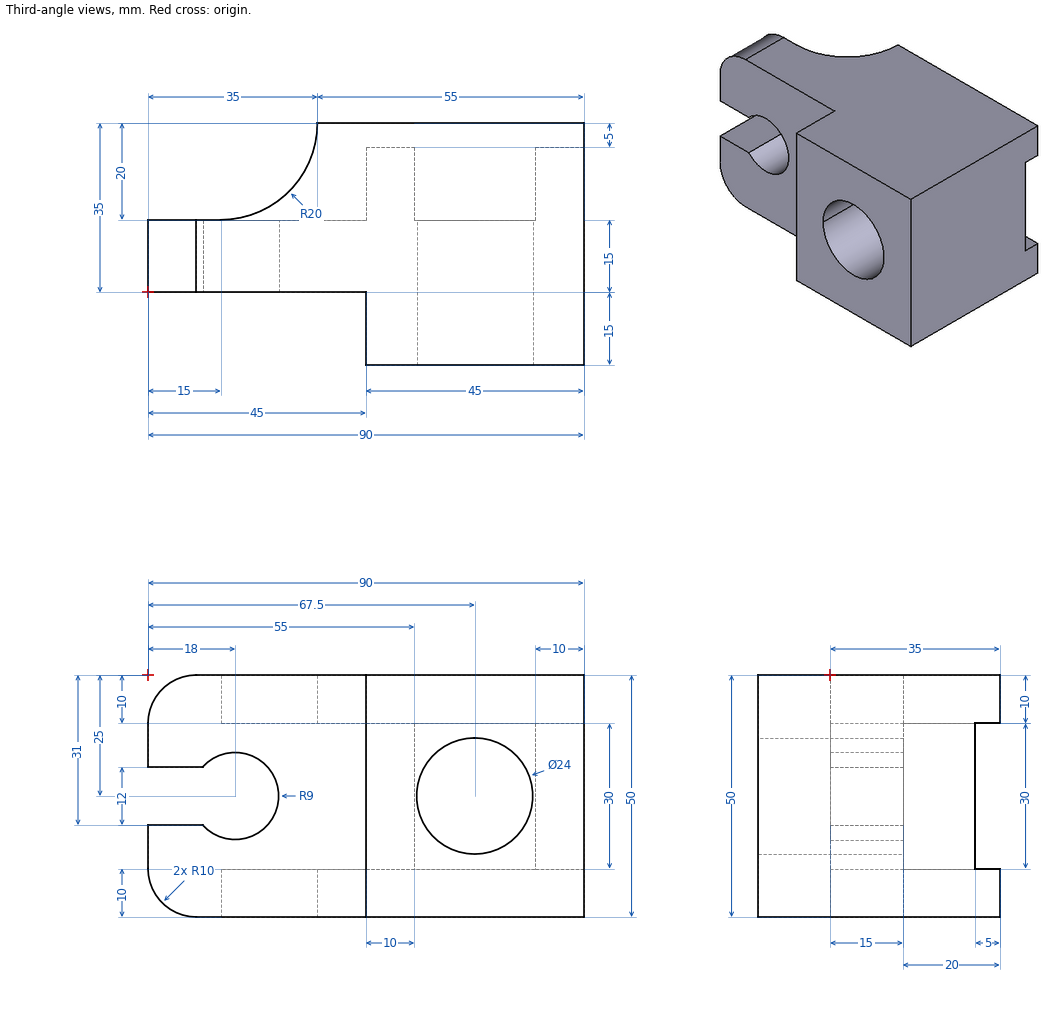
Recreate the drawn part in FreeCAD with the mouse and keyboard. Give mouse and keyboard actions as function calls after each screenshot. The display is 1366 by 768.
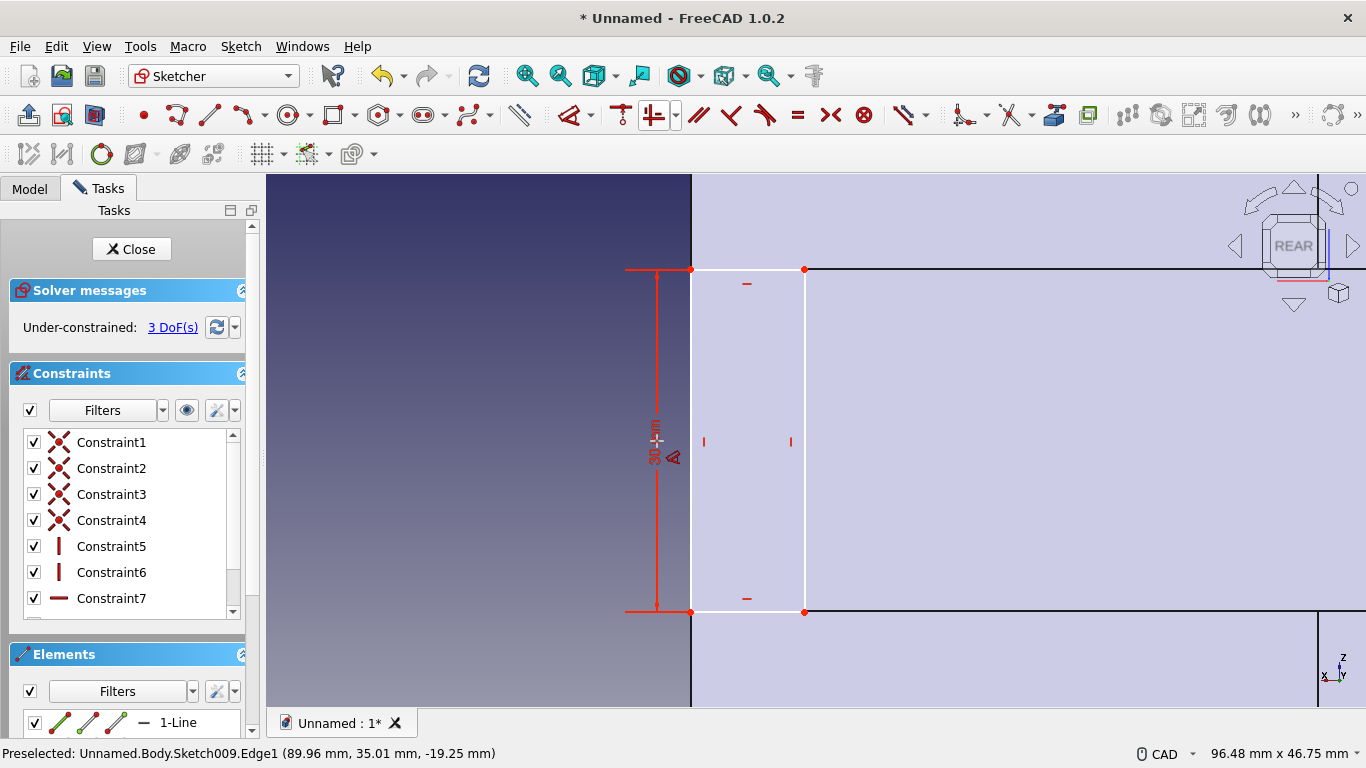
click(725, 612)
click(748, 646)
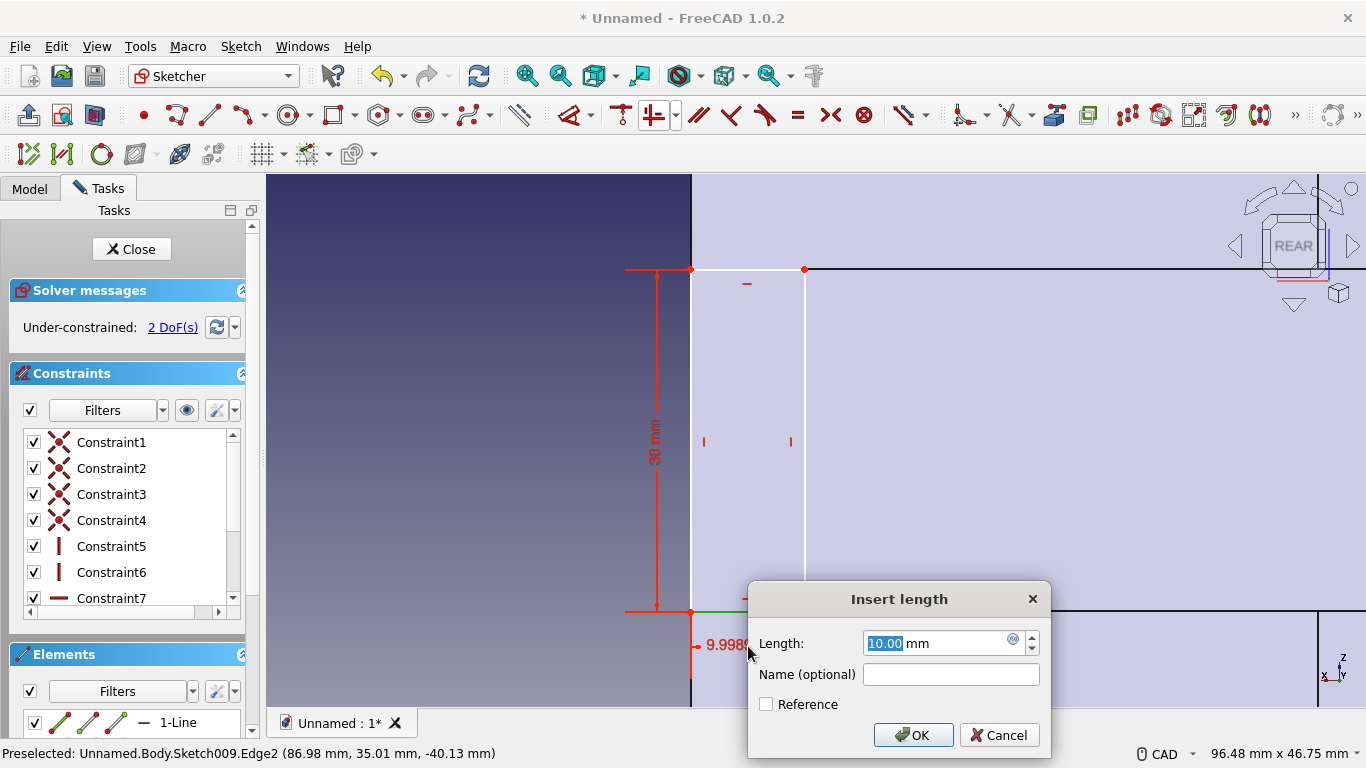
text(10)
key(Return)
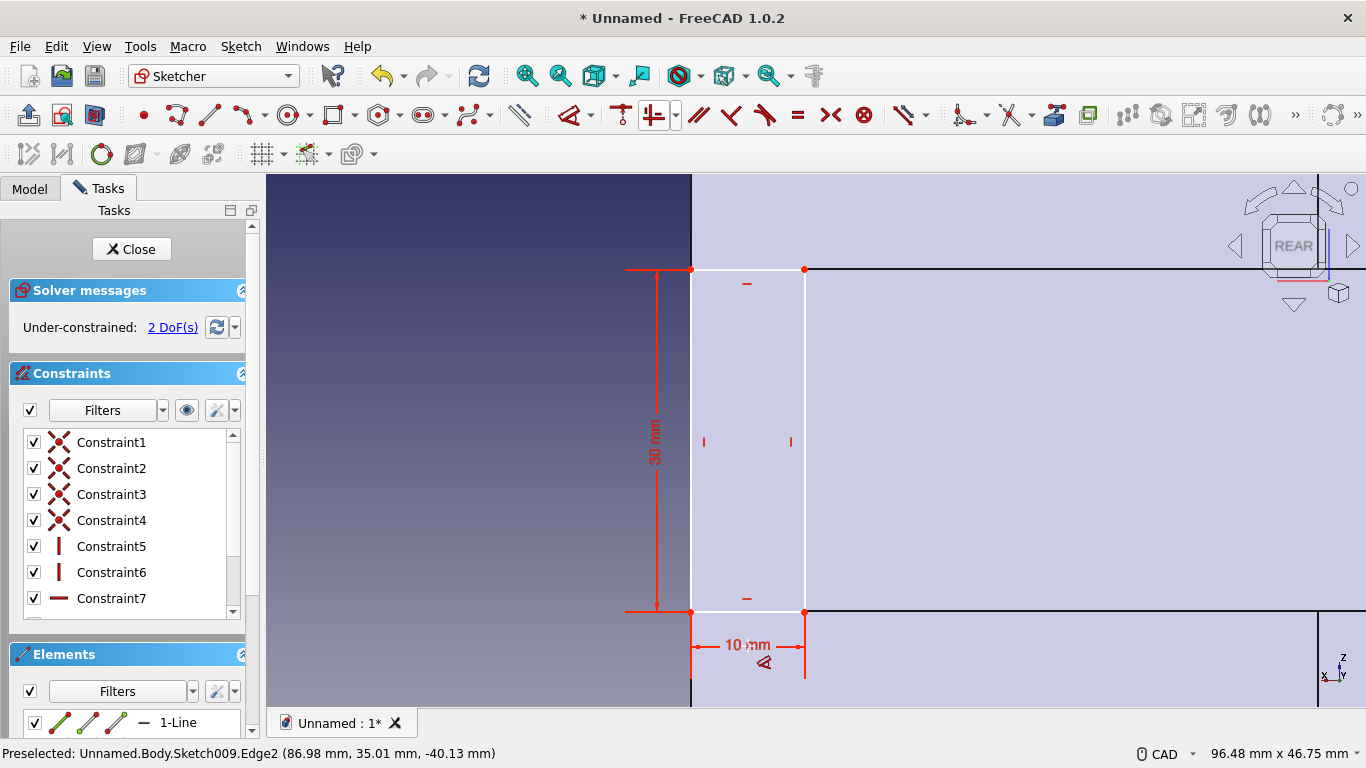
click(691, 270)
click(946, 304)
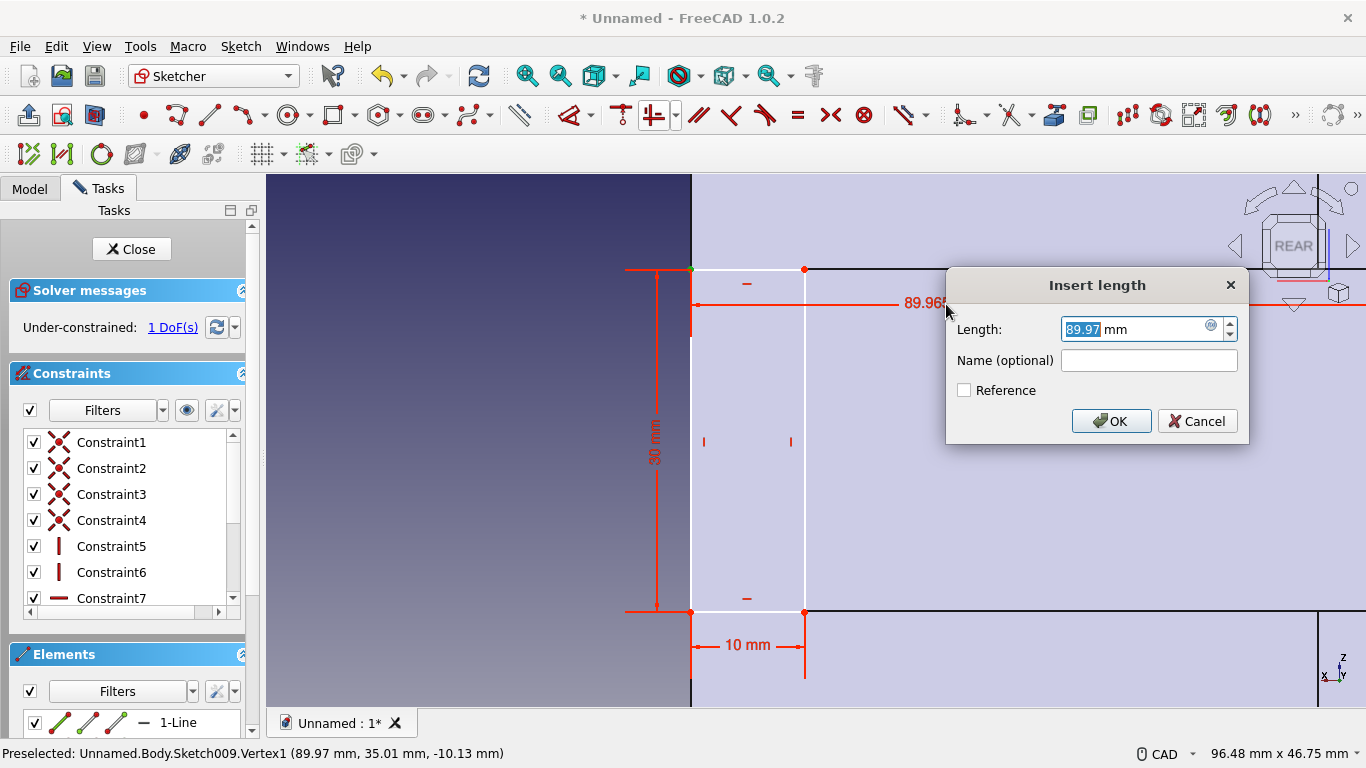
text(90)
key(Return)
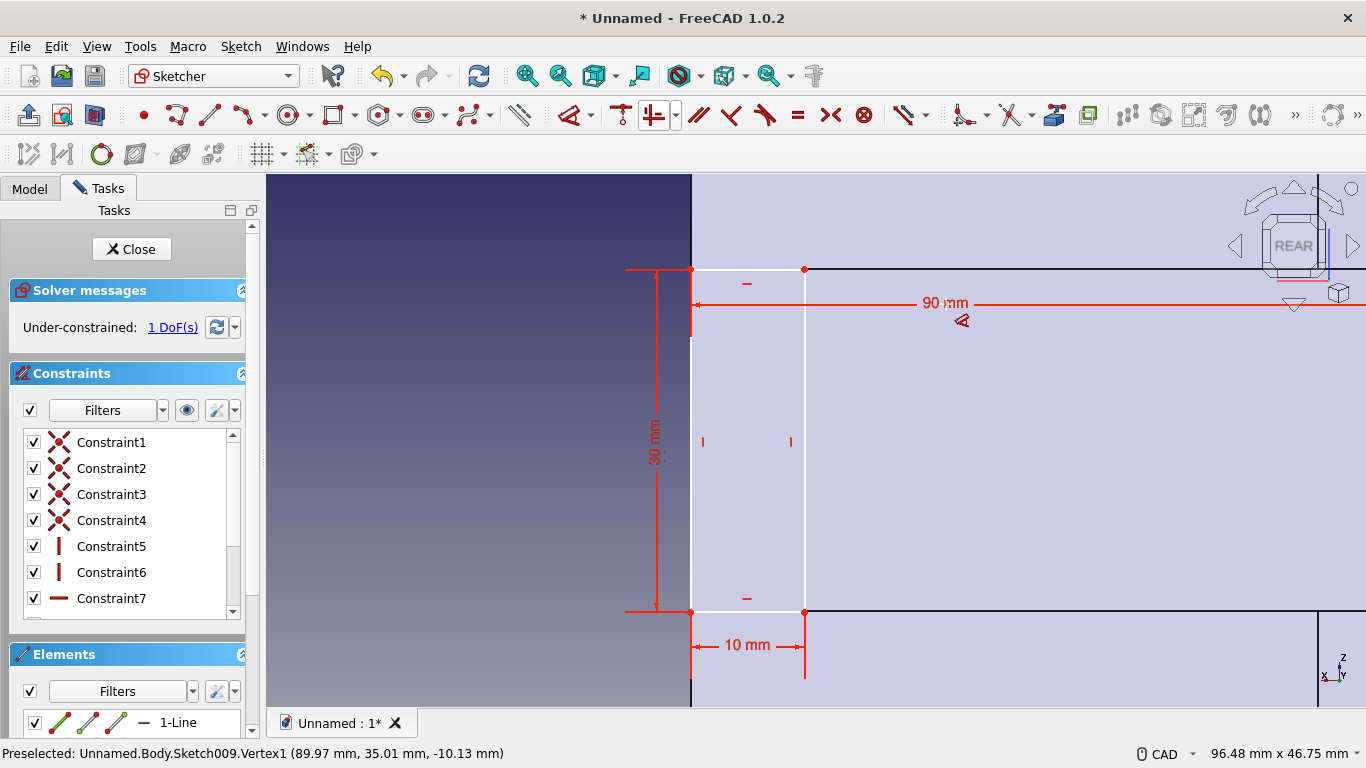
click(691, 270)
click(657, 236)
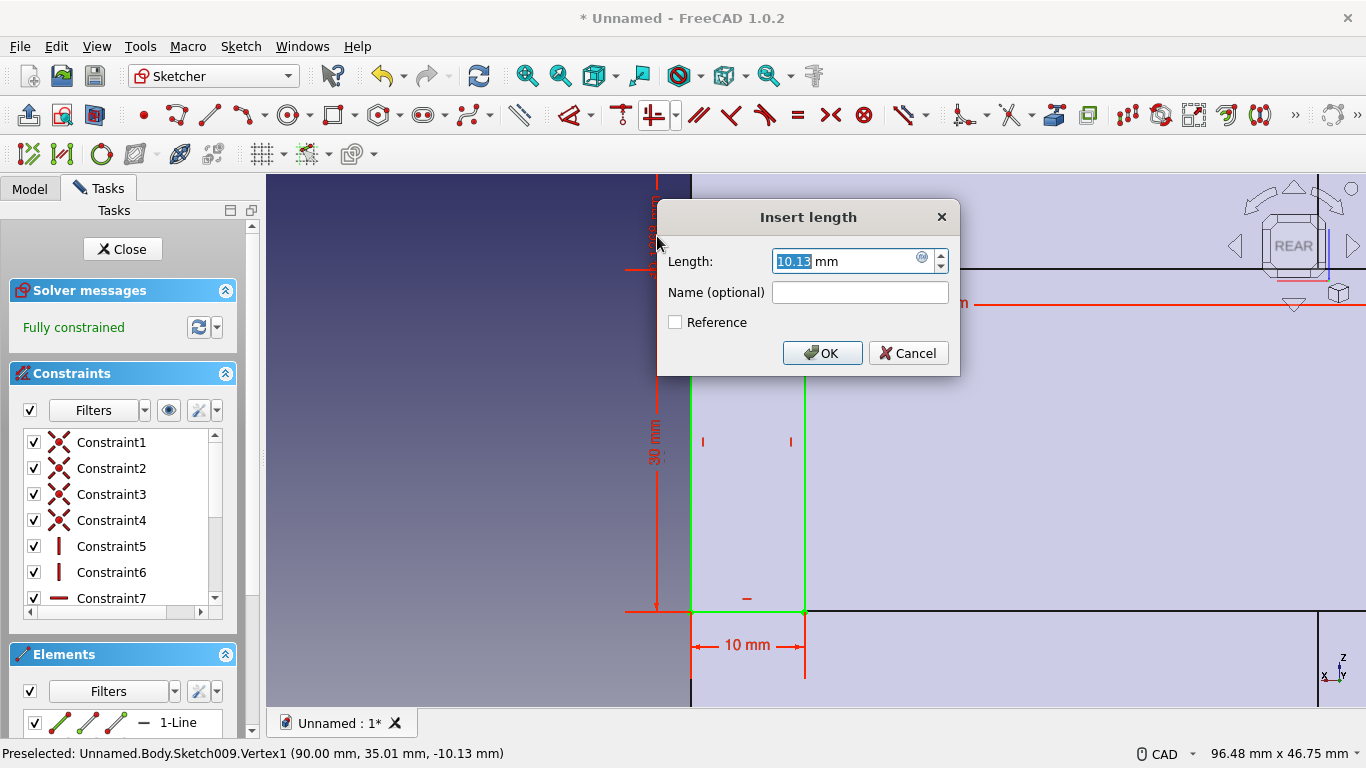
text(10)
key(Return)
key(Escape)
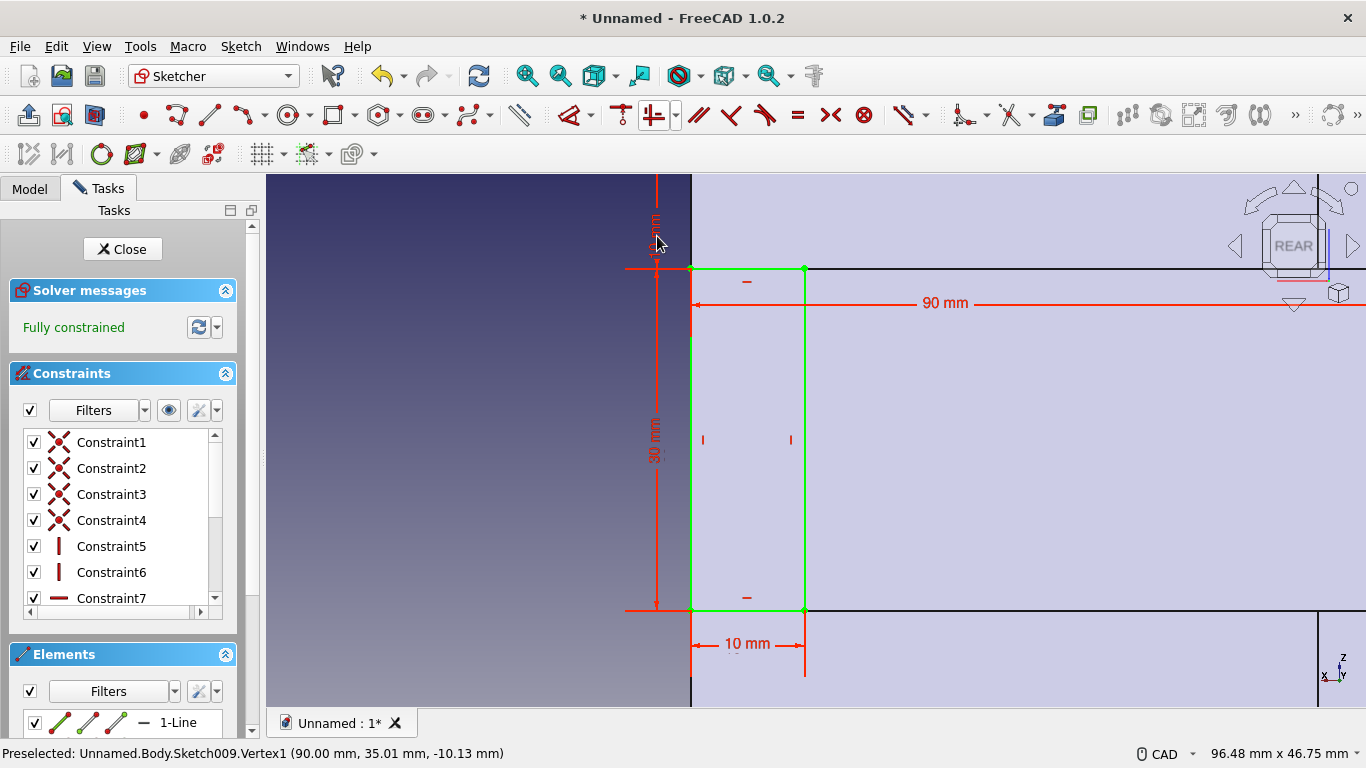
click(123, 249)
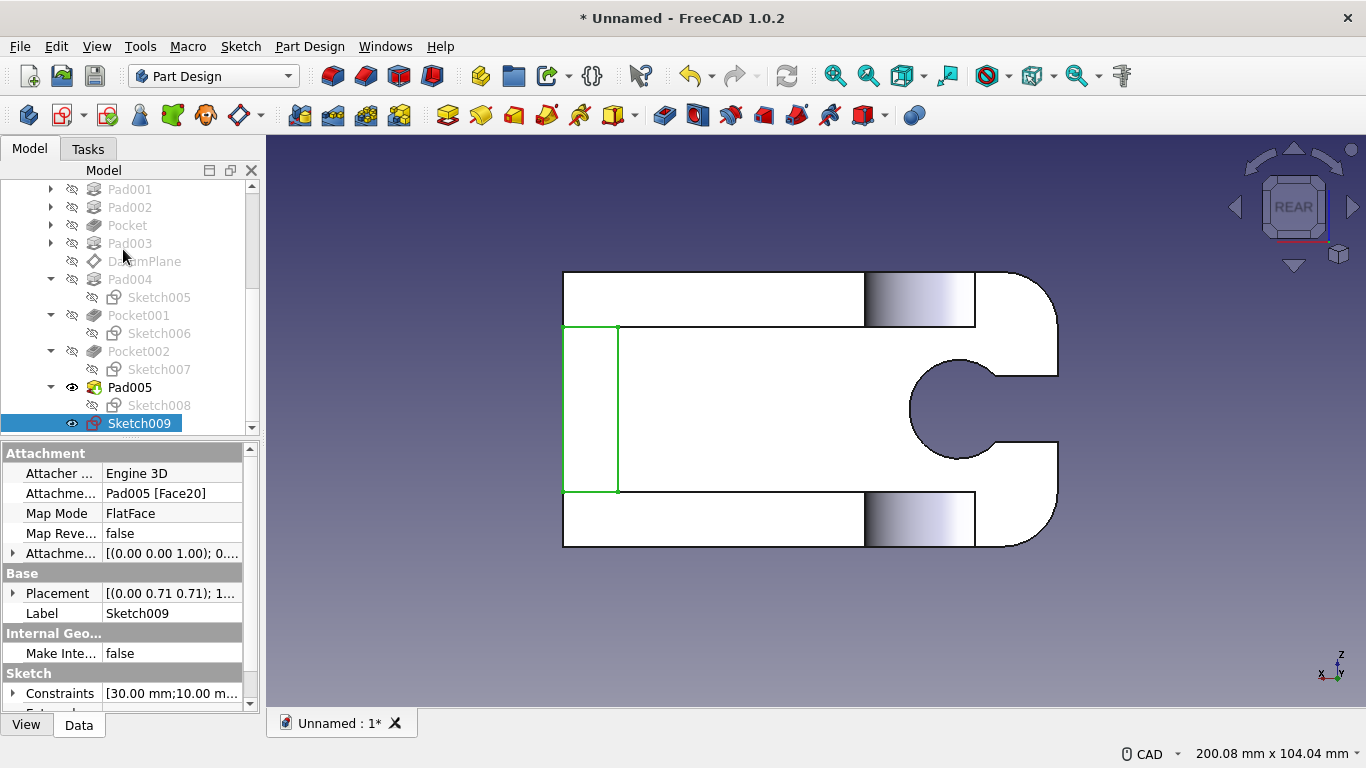
click(665, 116)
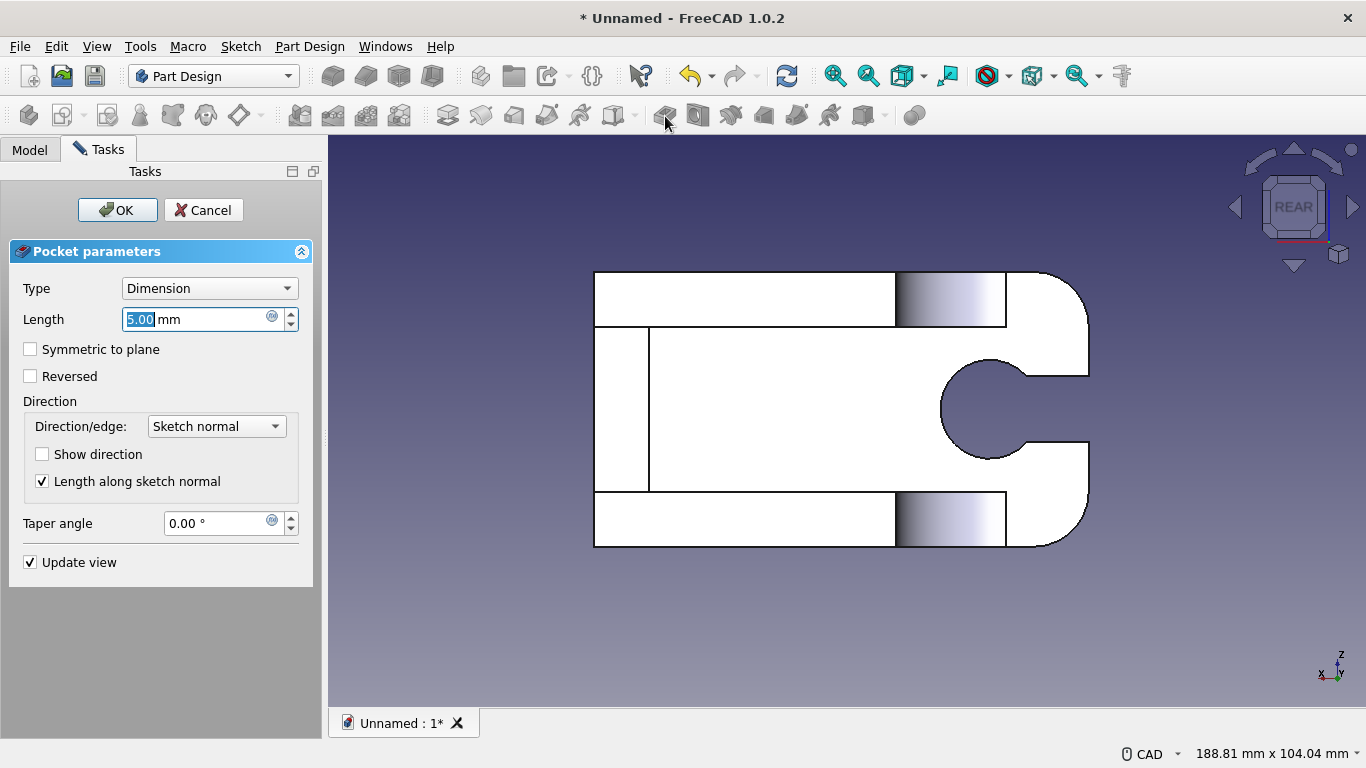
text(5)
key(Tab)